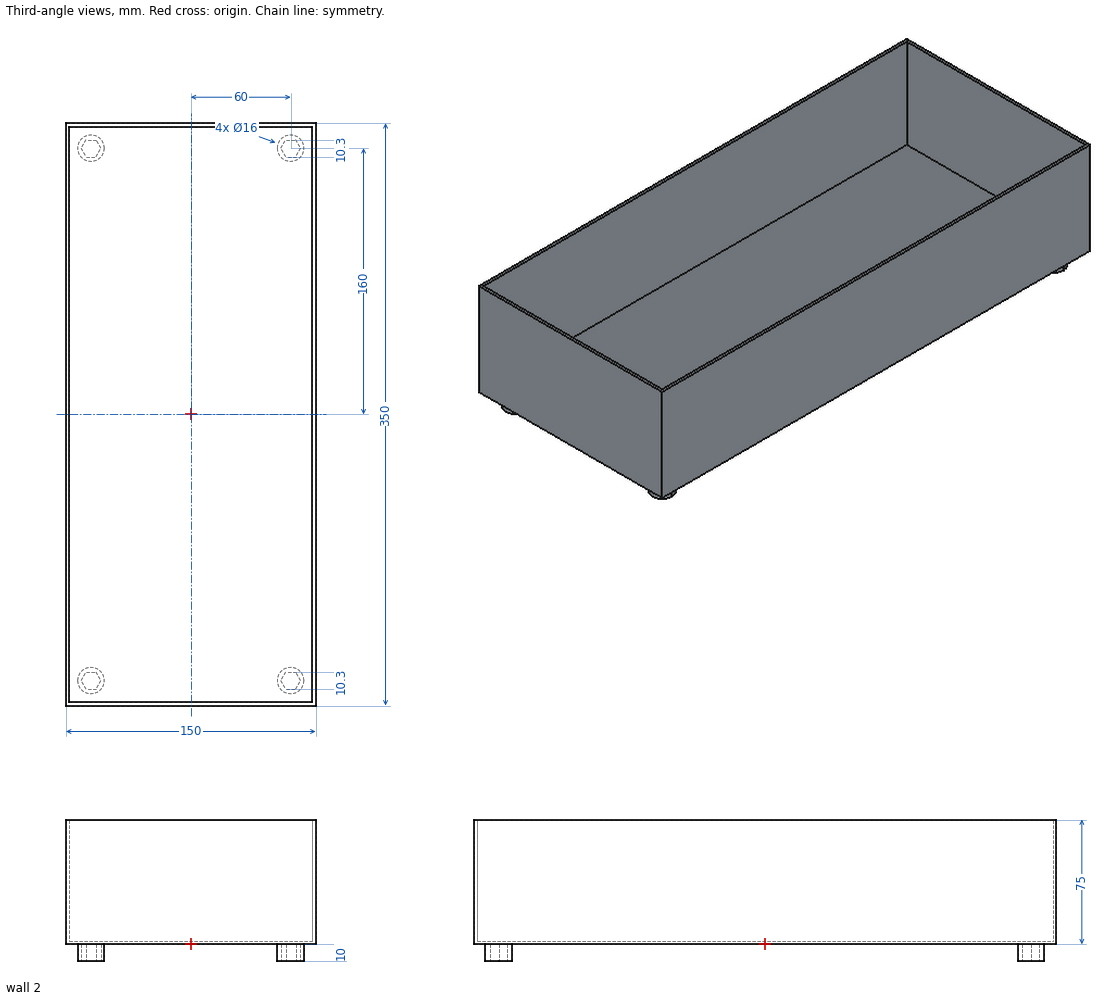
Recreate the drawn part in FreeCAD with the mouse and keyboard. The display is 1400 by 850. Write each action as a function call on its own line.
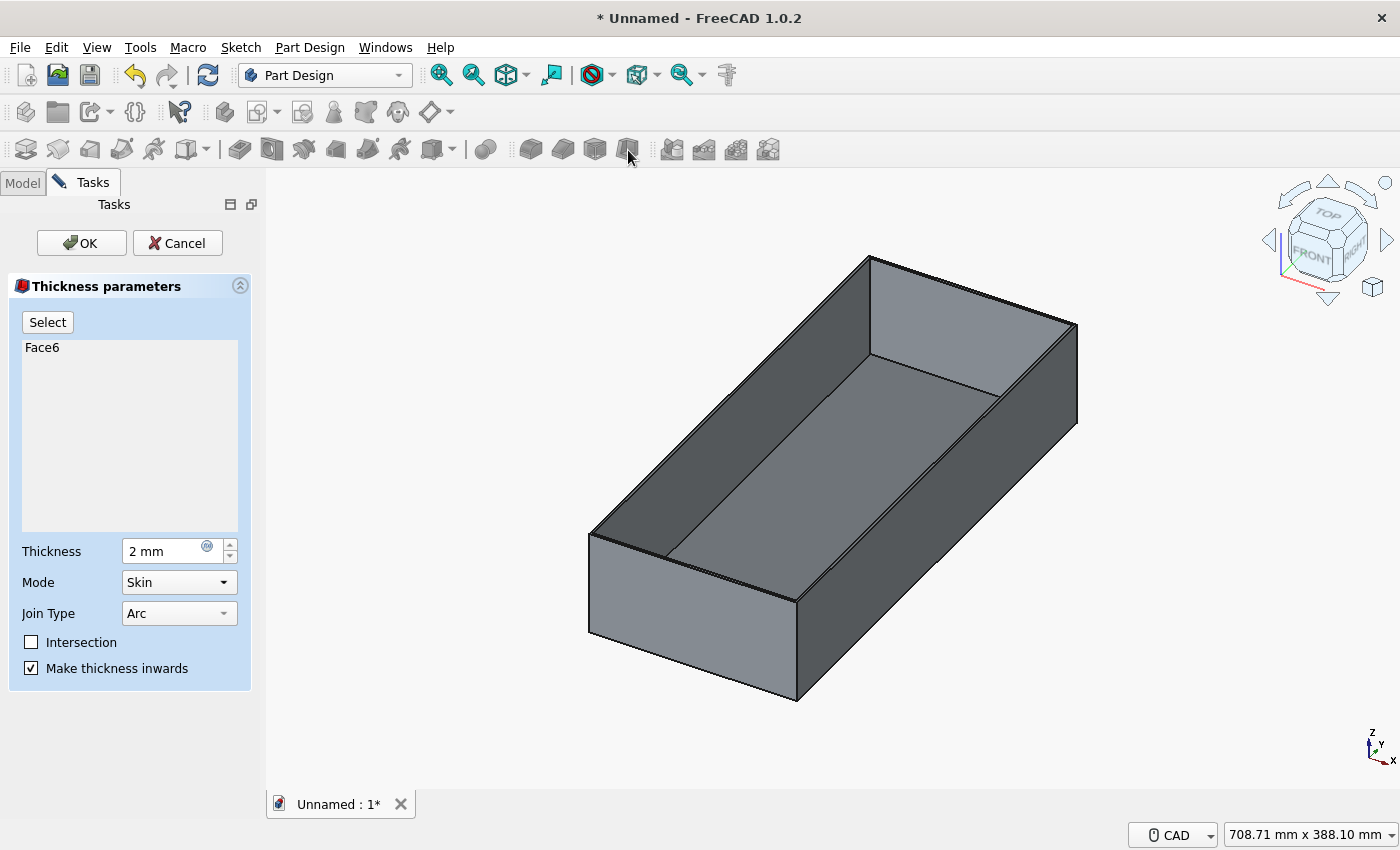
click(180, 614)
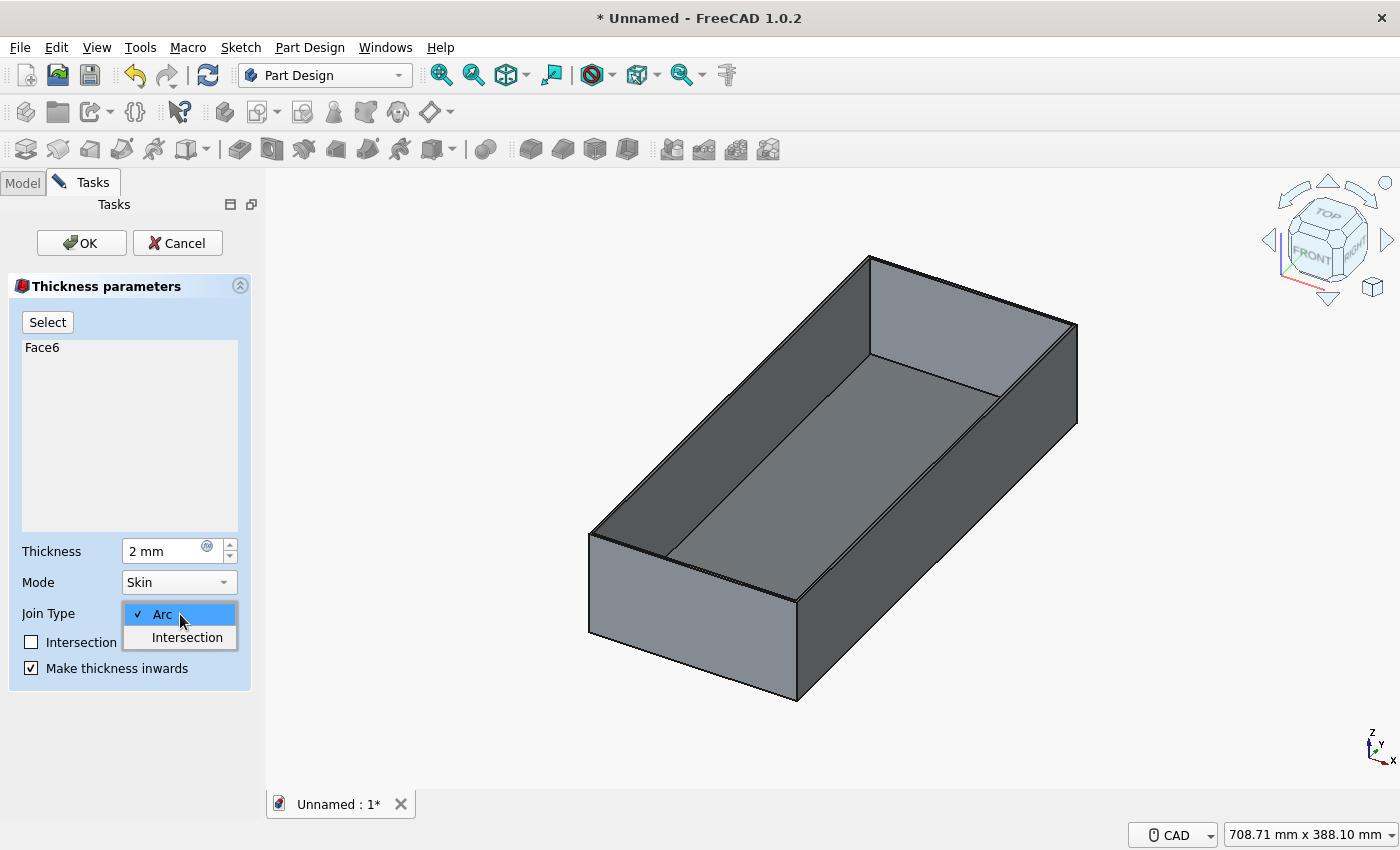
click(179, 638)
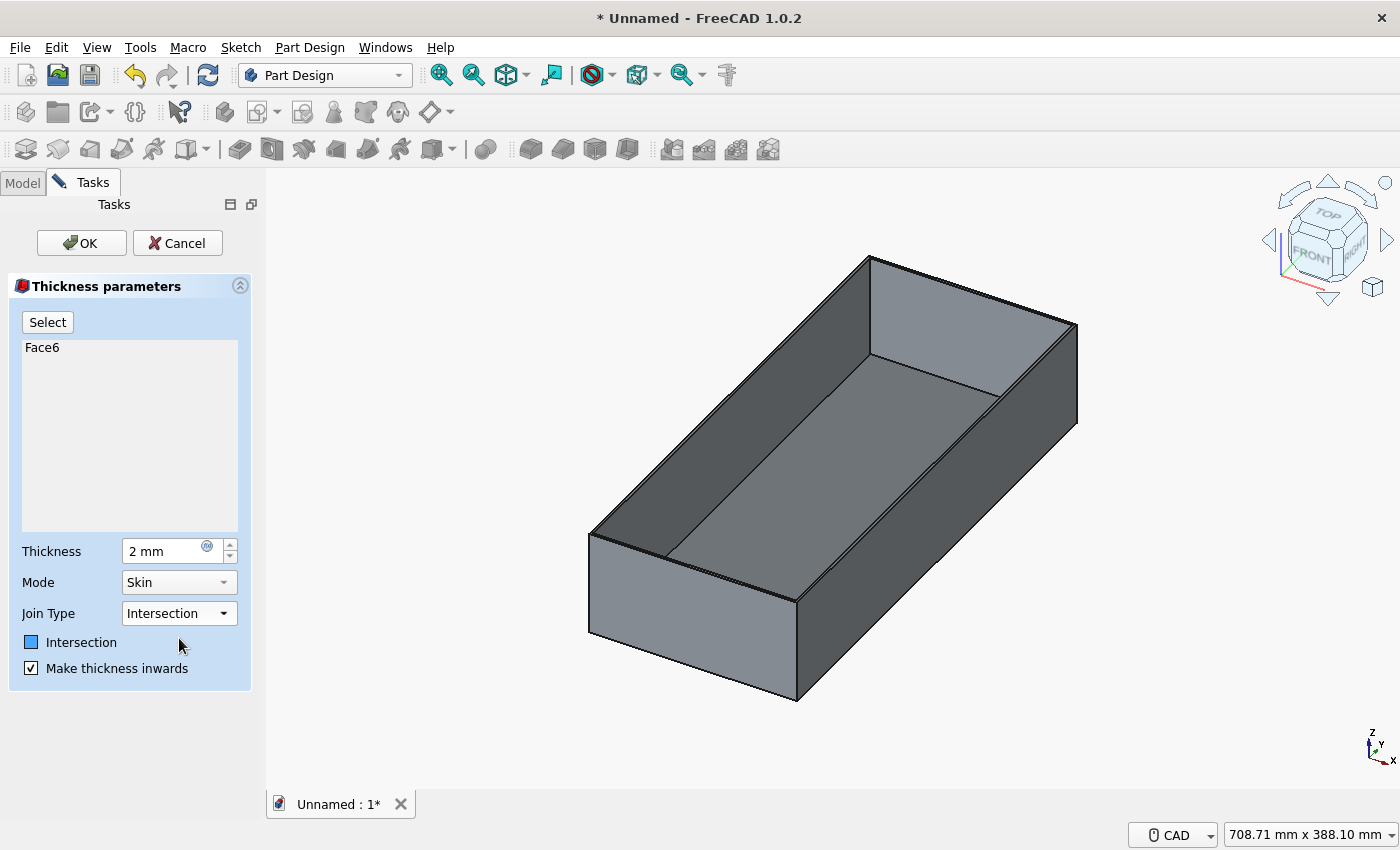
click(82, 243)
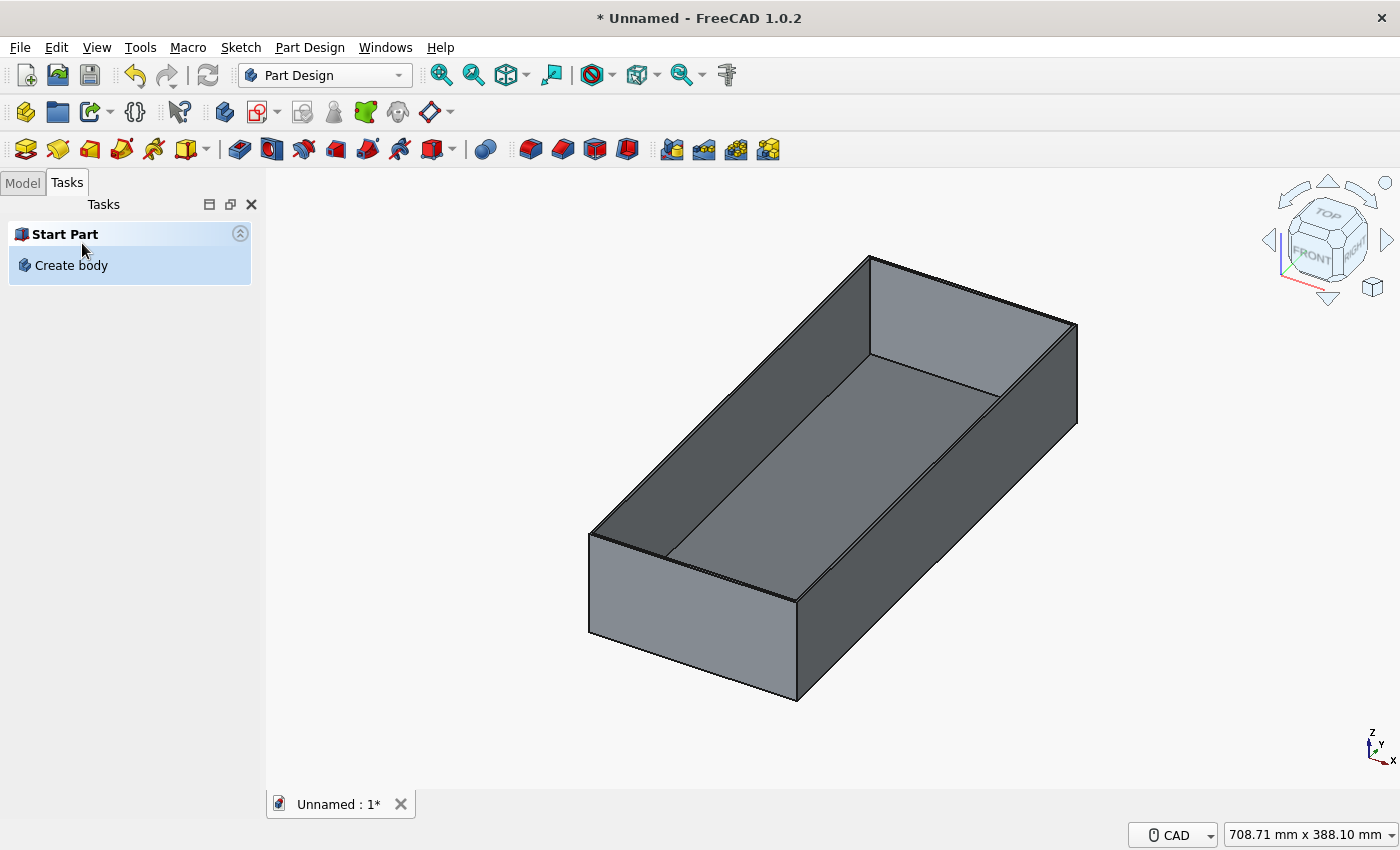
click(258, 112)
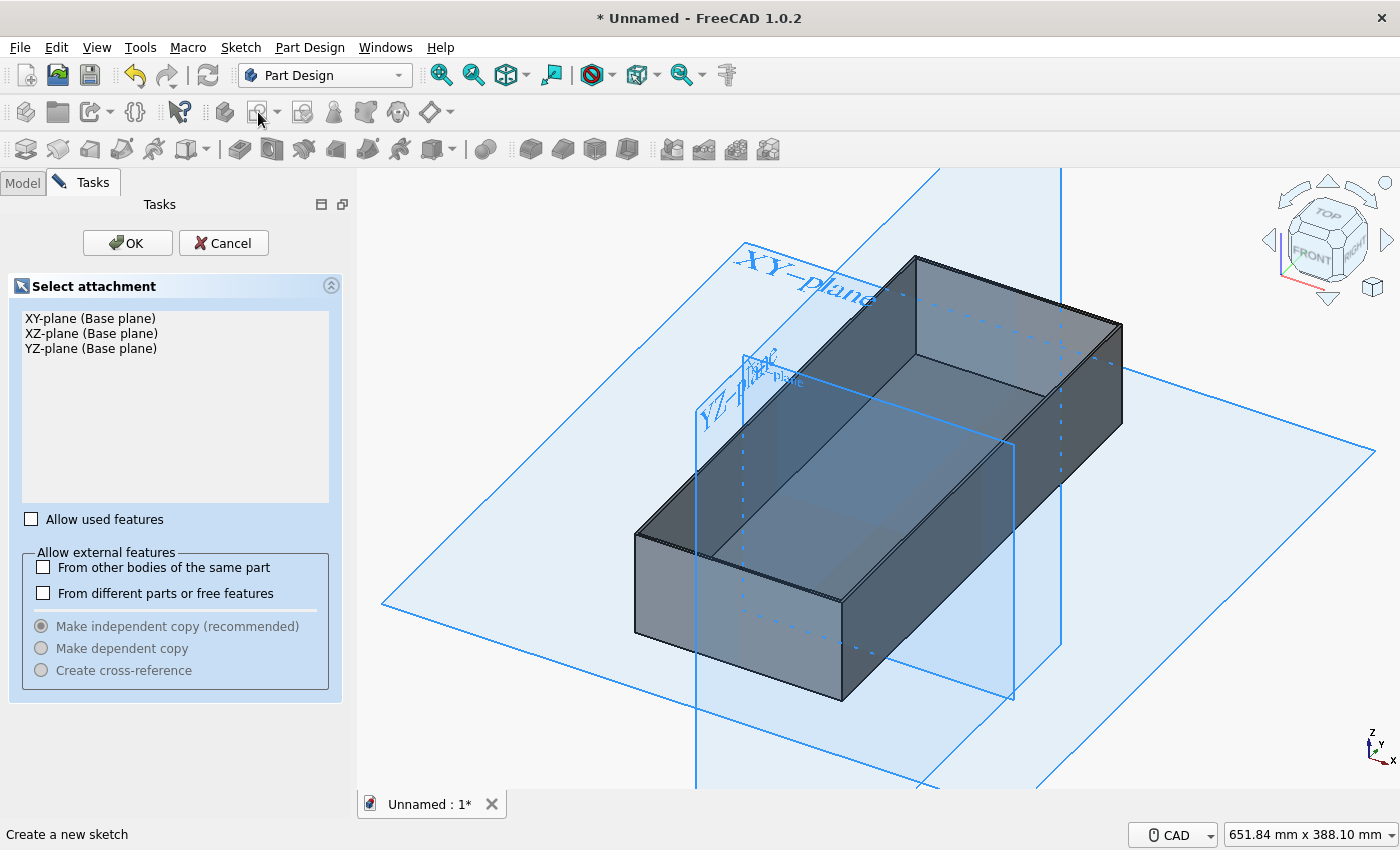
click(82, 318)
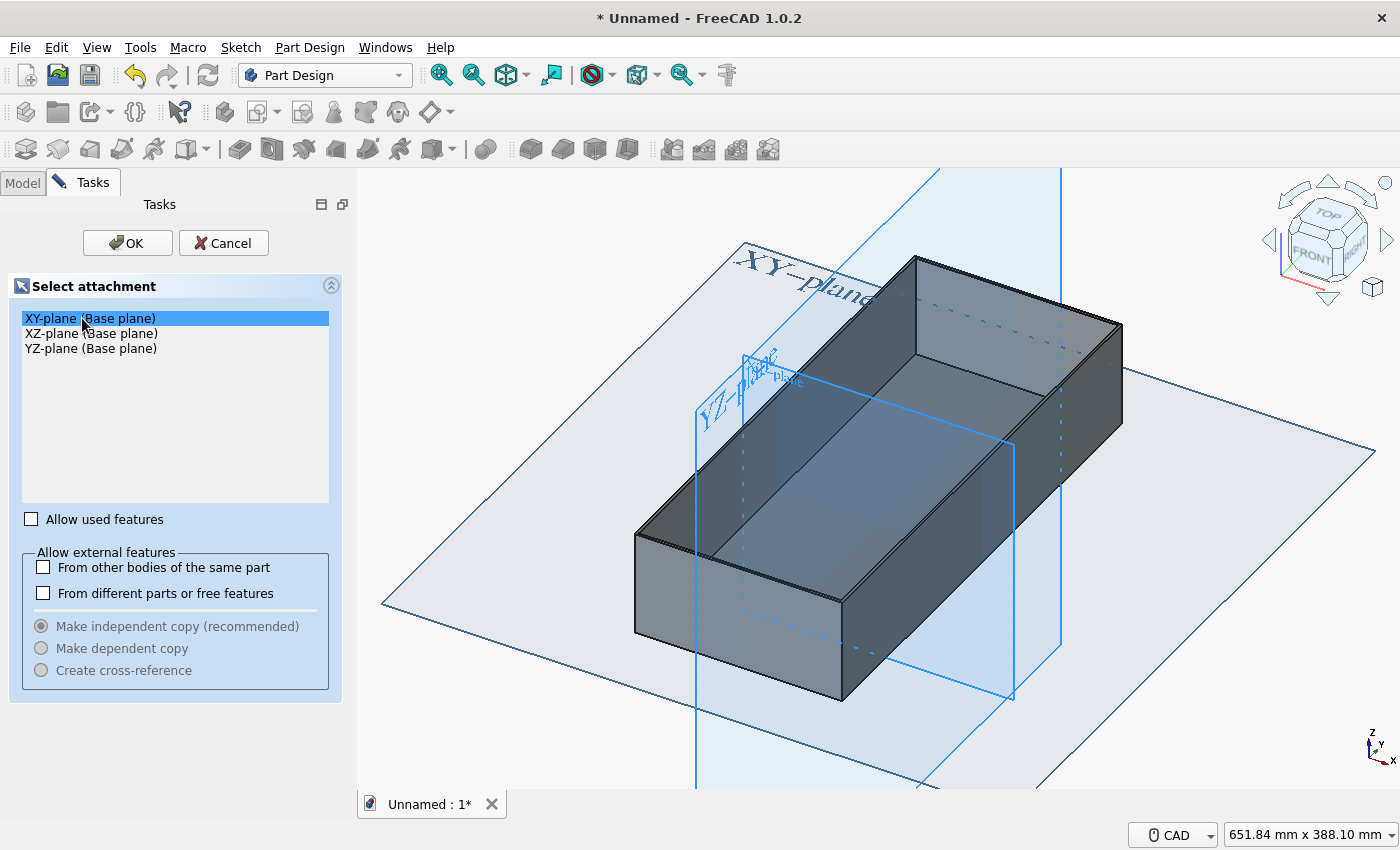
click(128, 243)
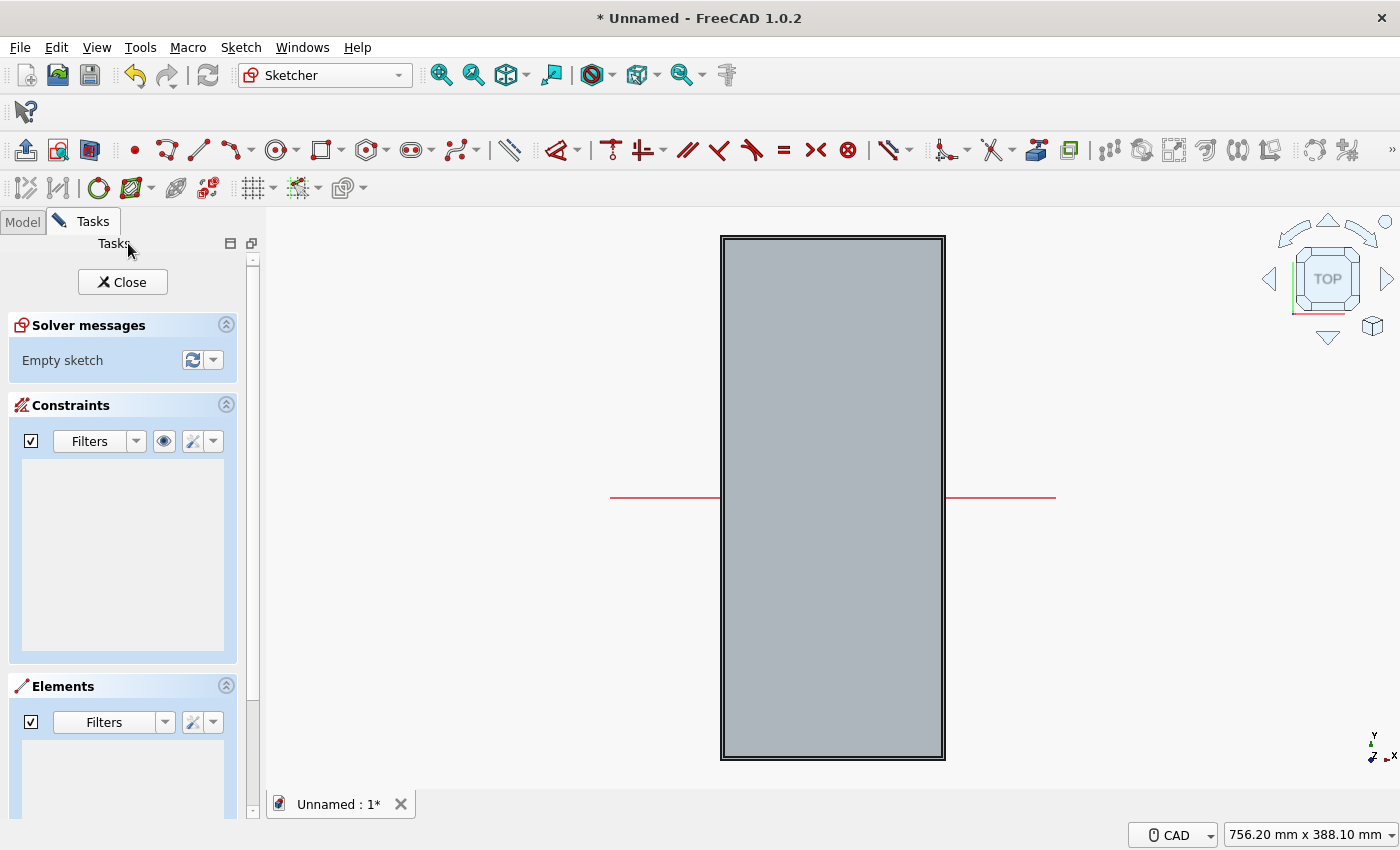
click(90, 150)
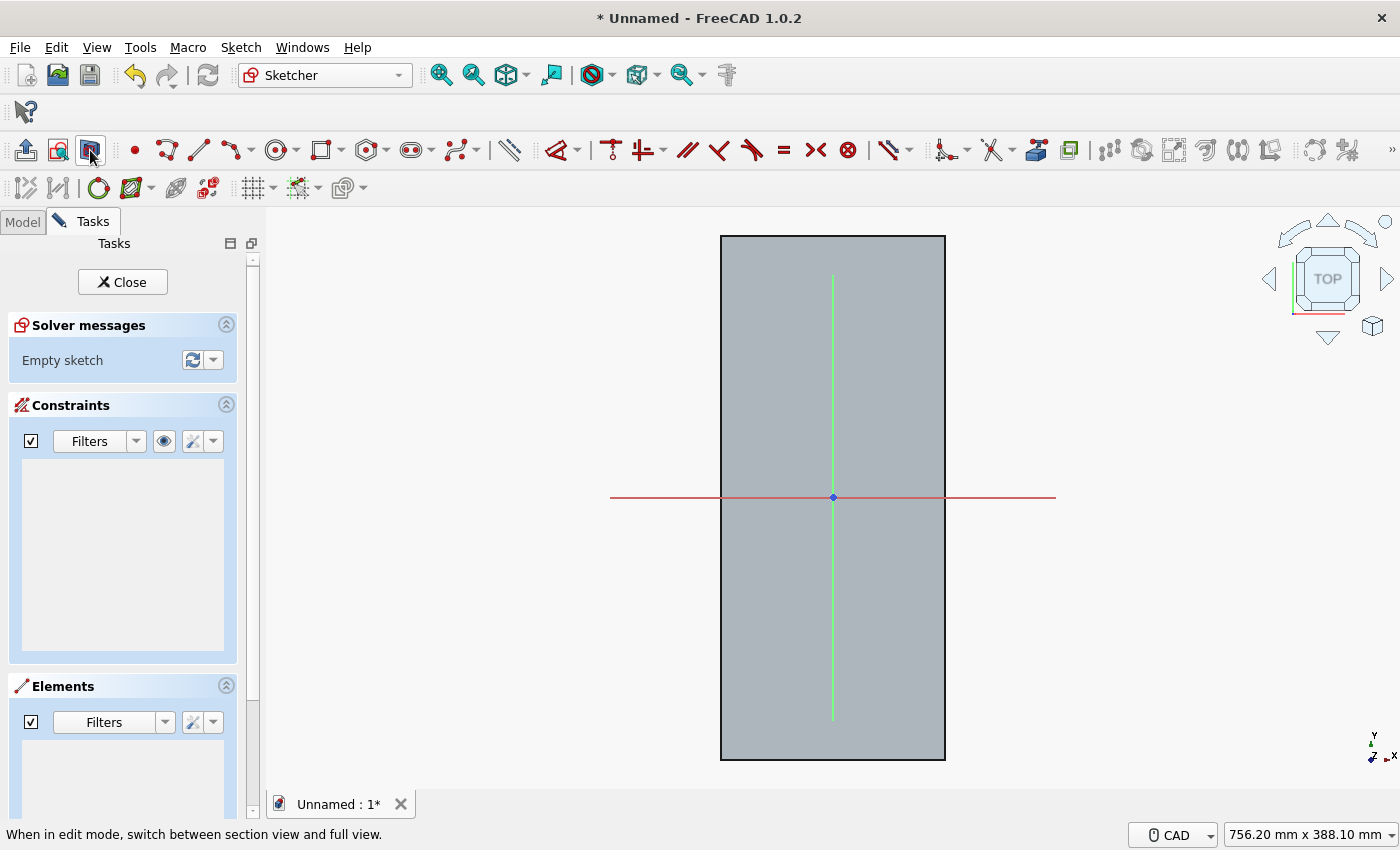
scroll(625, 498, down, 2)